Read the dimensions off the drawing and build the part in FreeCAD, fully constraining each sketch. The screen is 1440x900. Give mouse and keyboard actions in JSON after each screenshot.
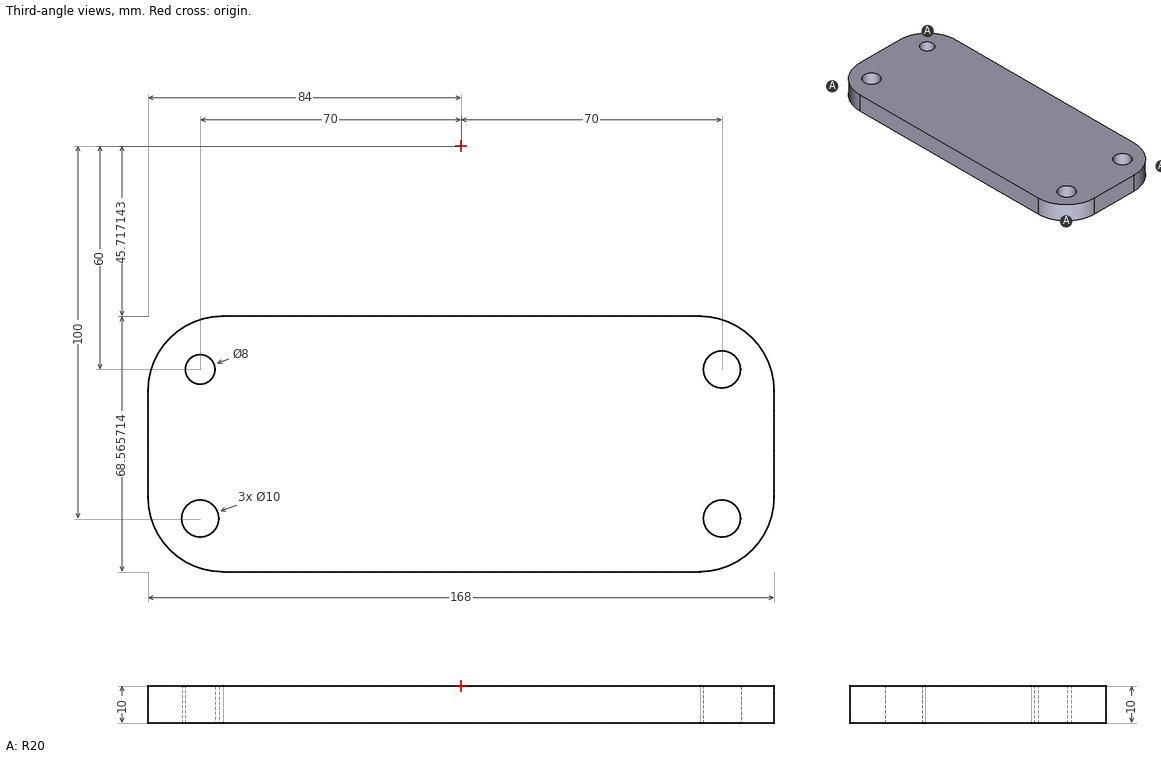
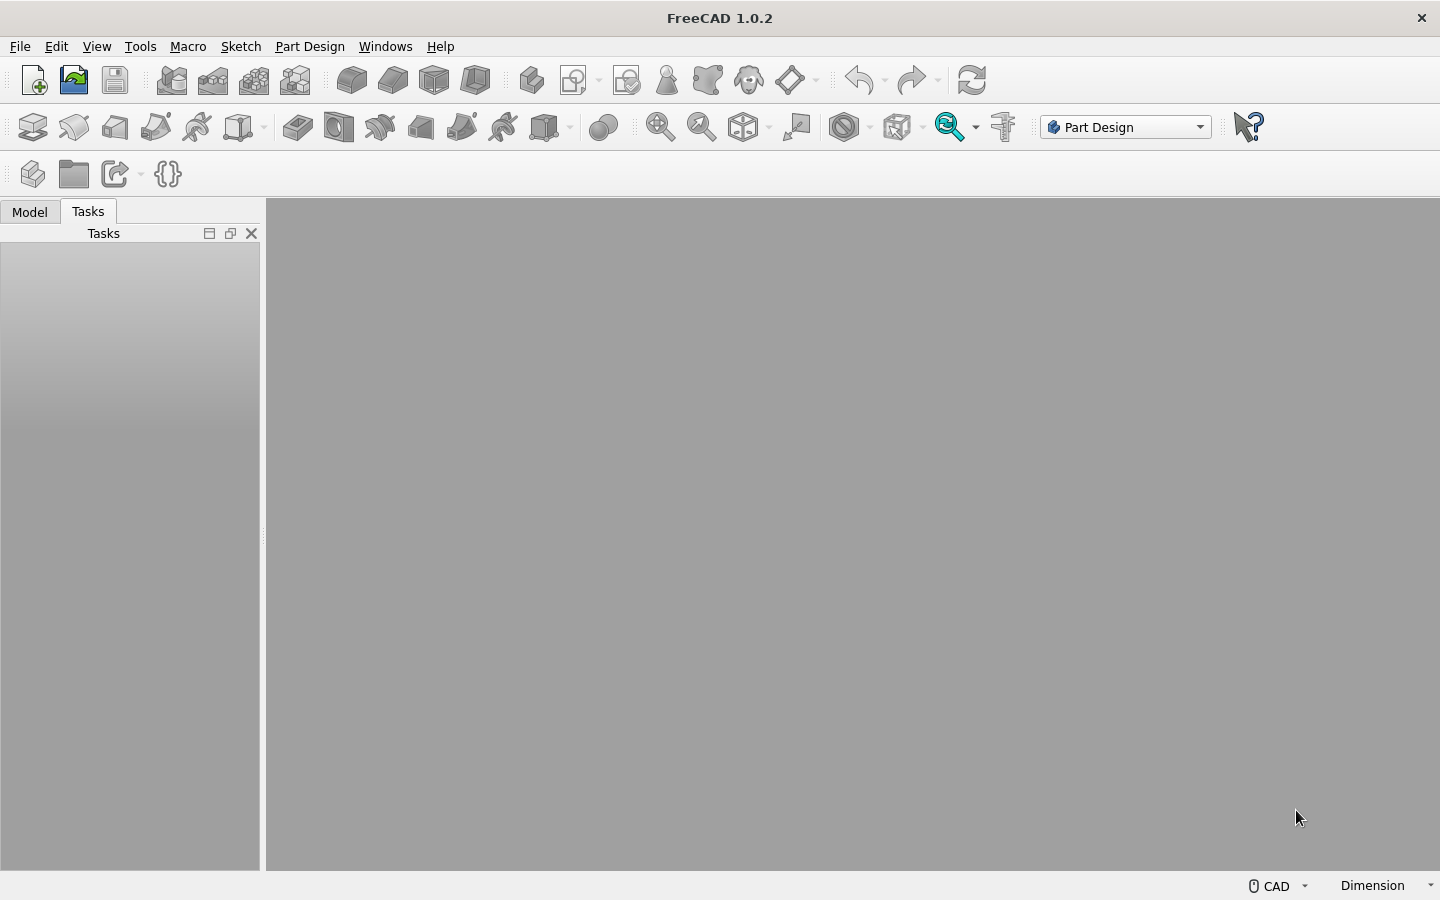
{"action": "left_click", "coordinate": [33, 80]}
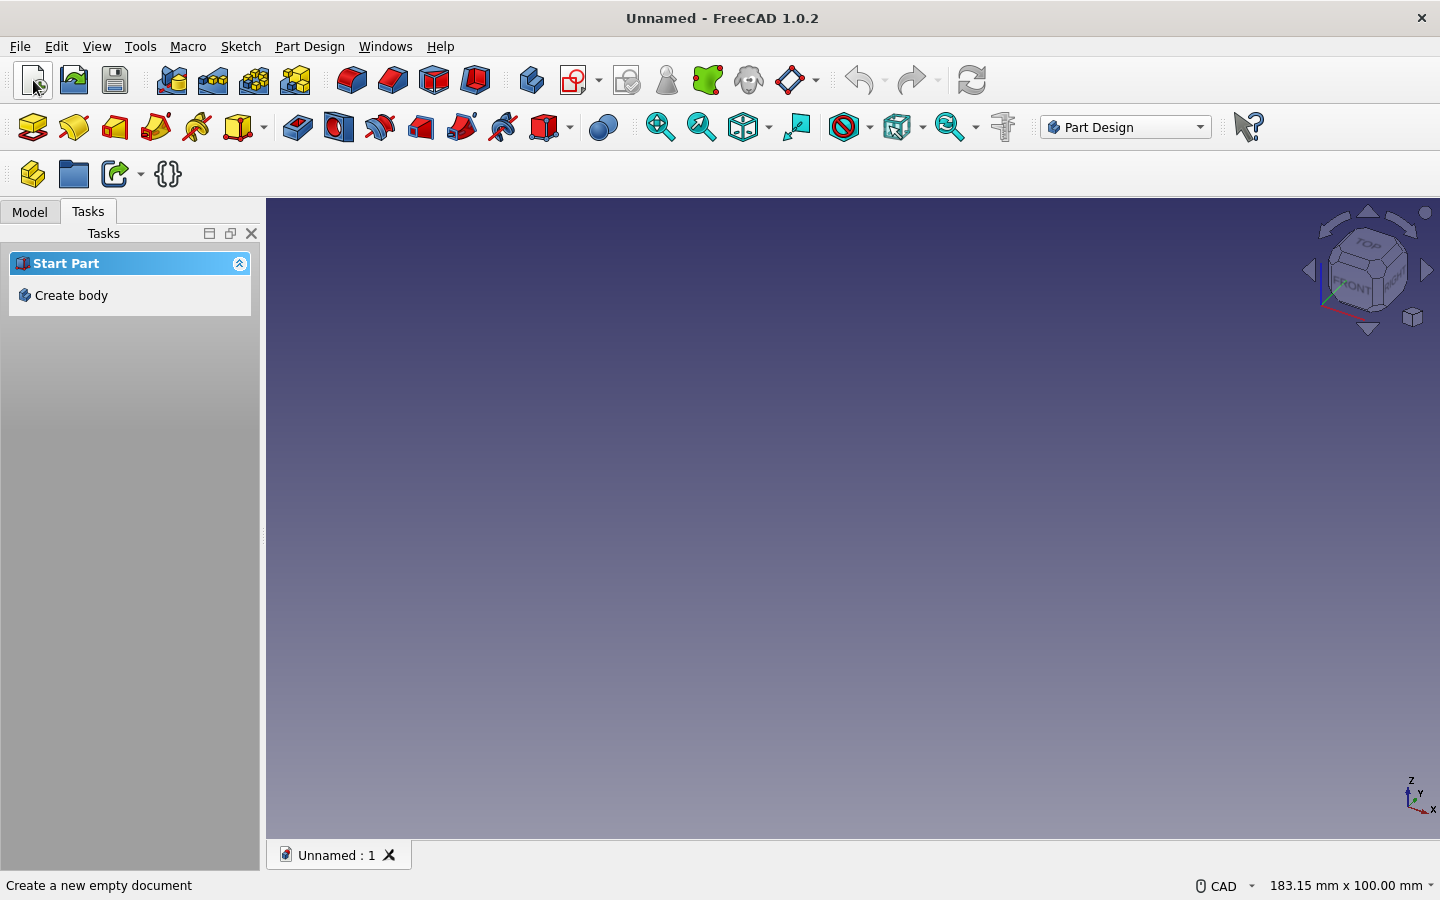
{"action": "left_click", "coordinate": [572, 80]}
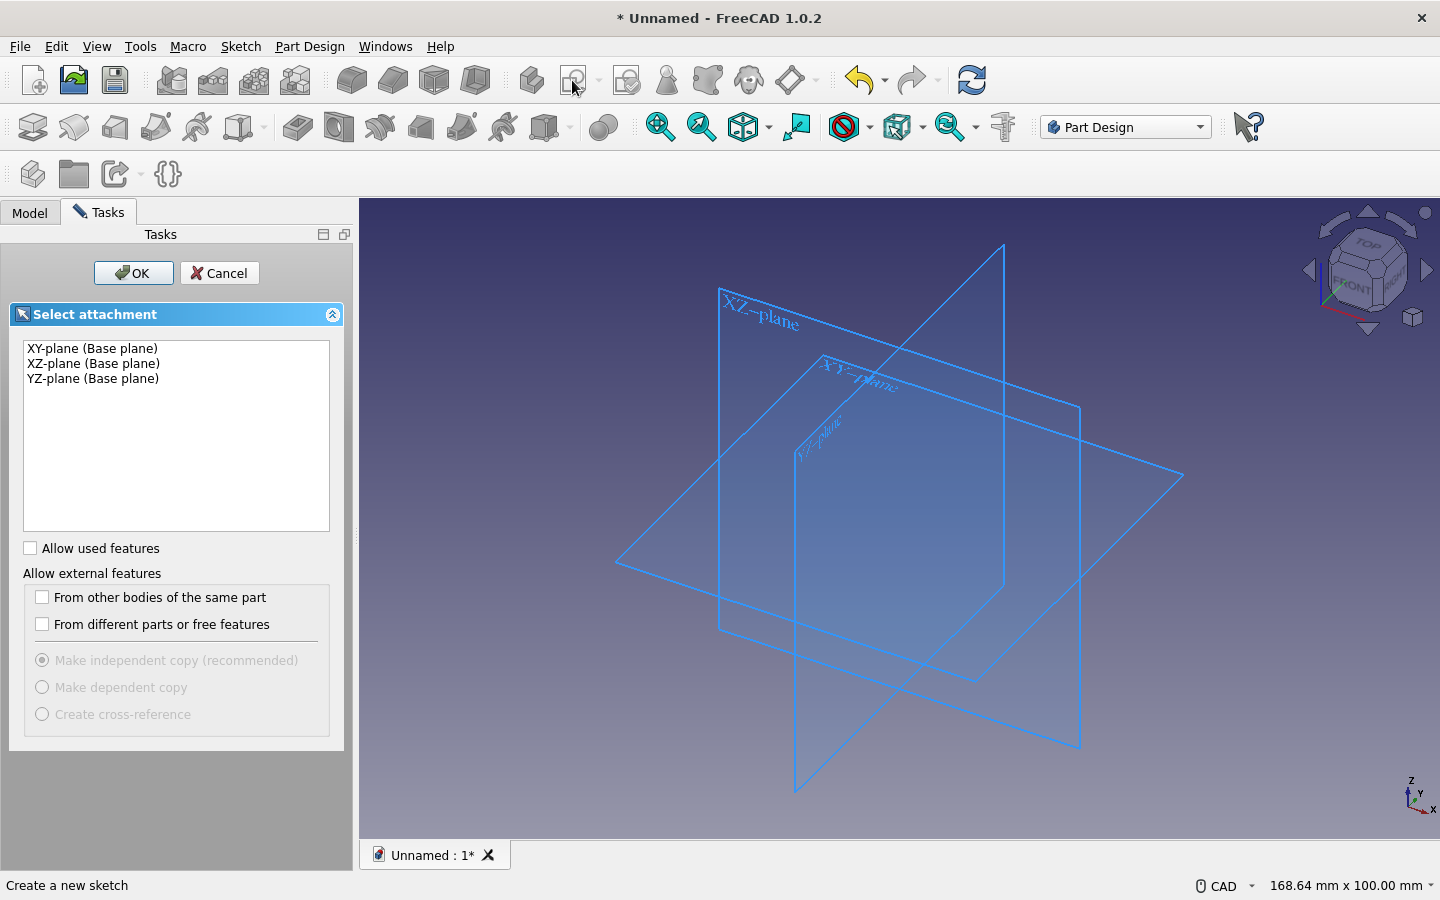
{"action": "left_click", "coordinate": [84, 348]}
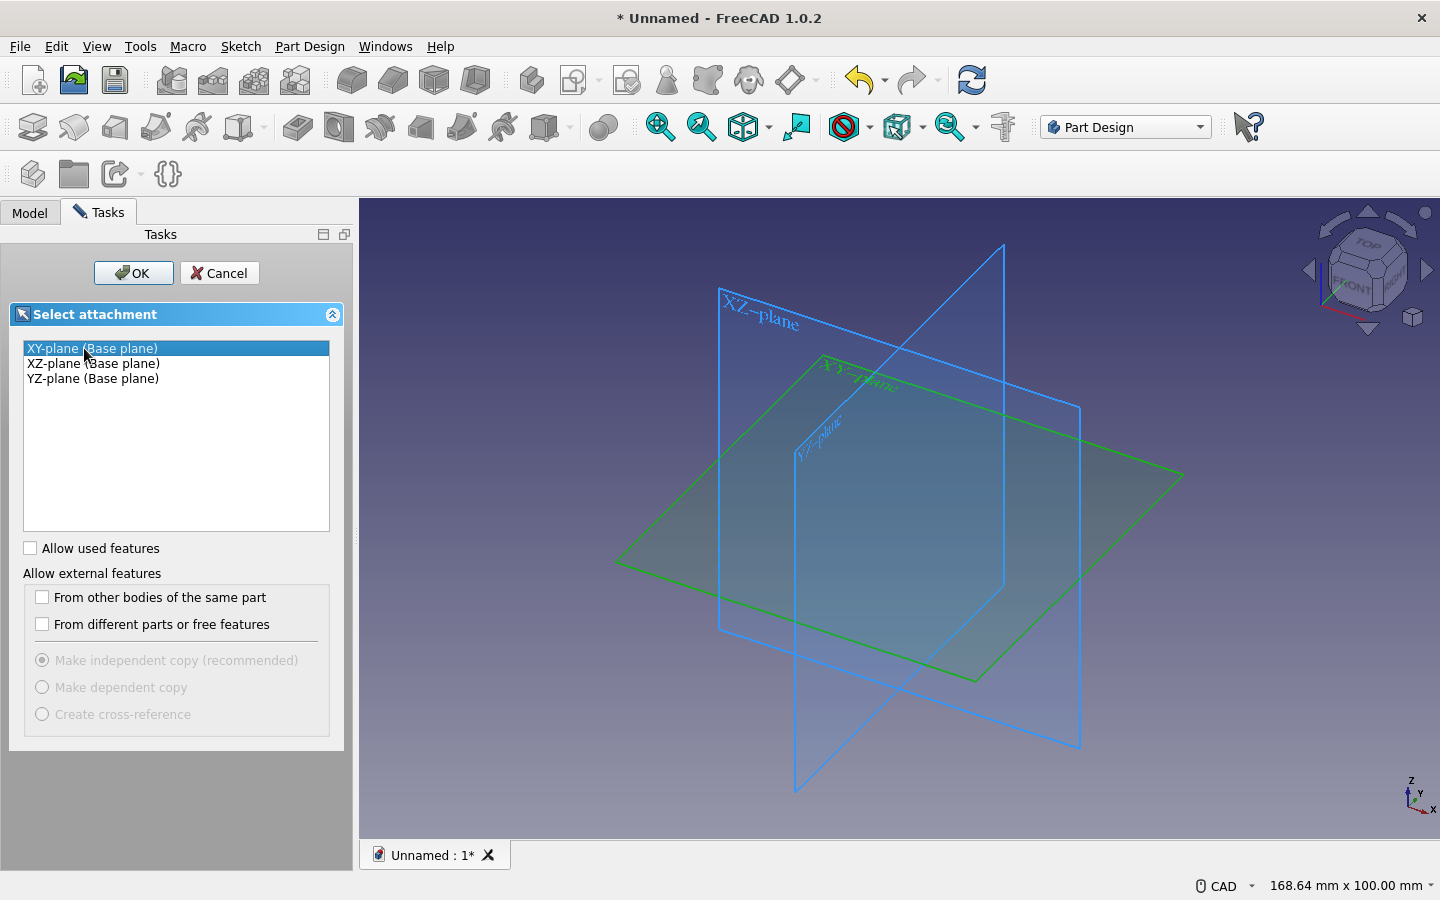
{"action": "left_click", "coordinate": [134, 273]}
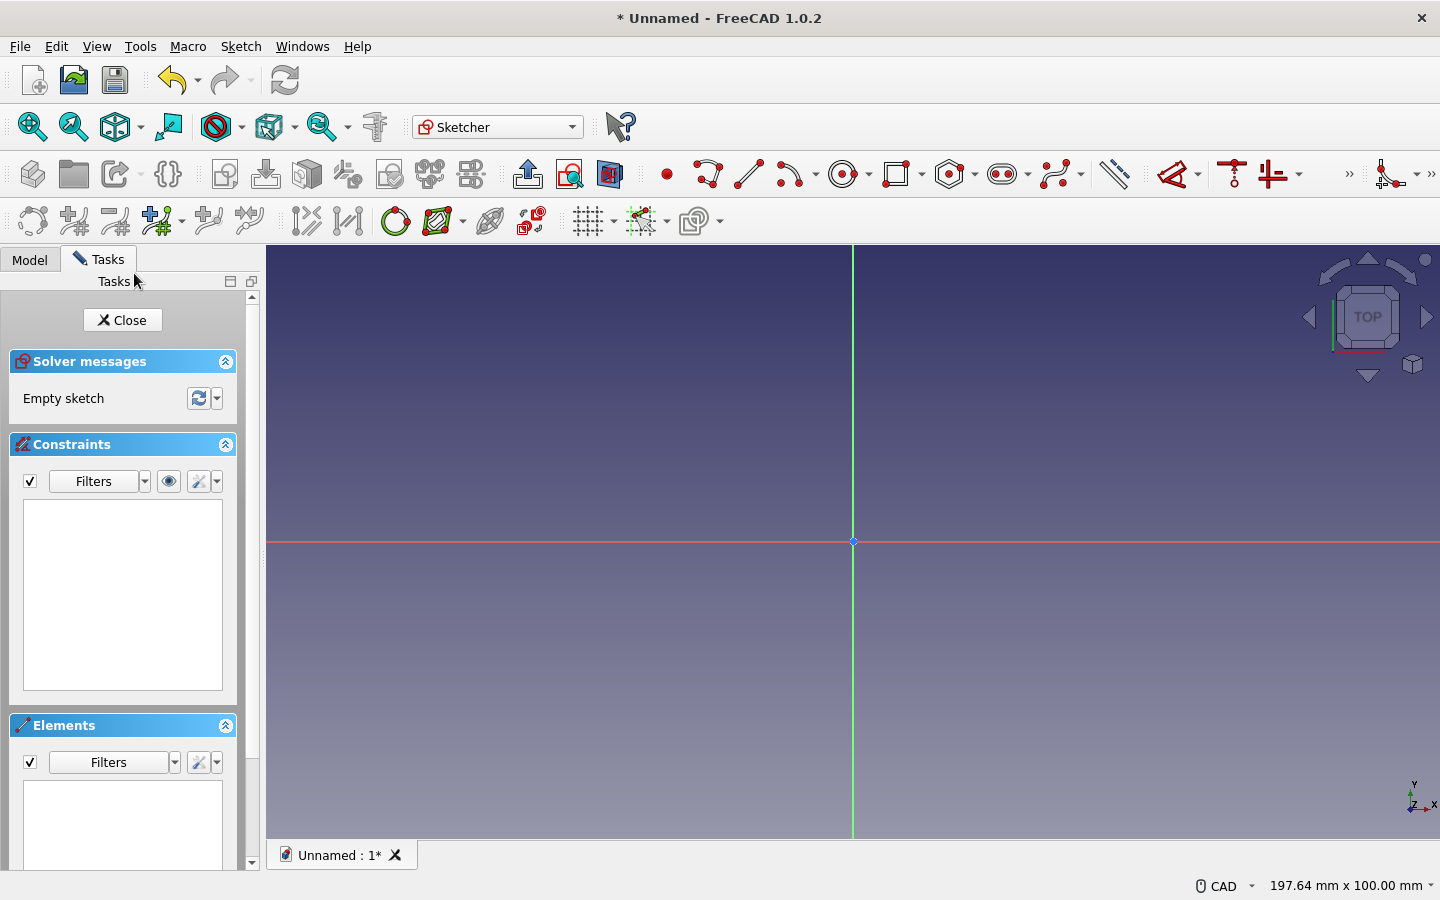
{"action": "scroll", "coordinate": [729, 273], "scroll_direction": "down", "scroll_amount": 4}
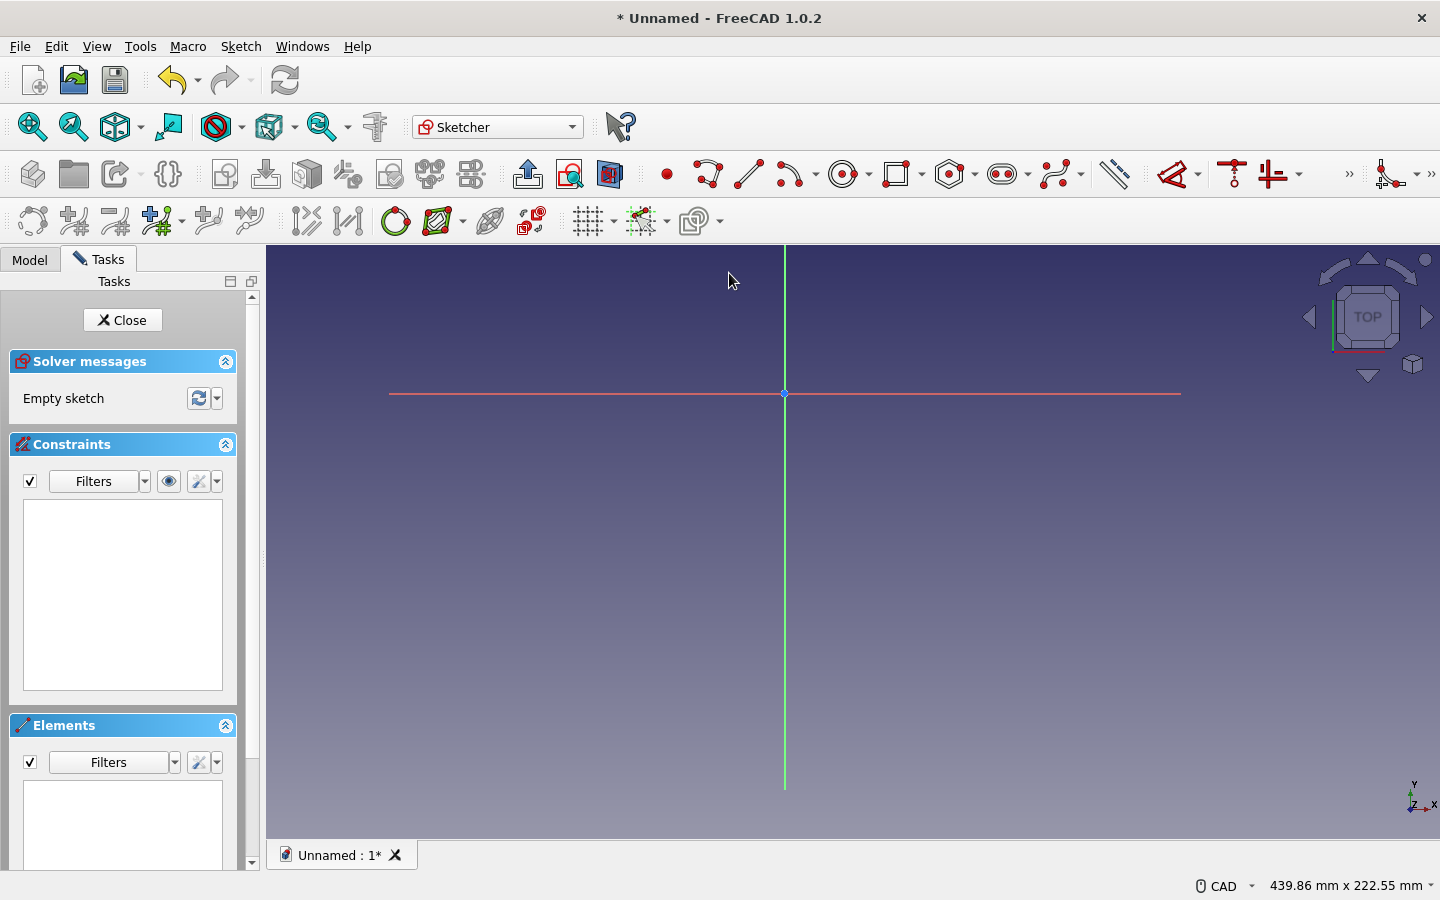
{"action": "left_click", "coordinate": [896, 174]}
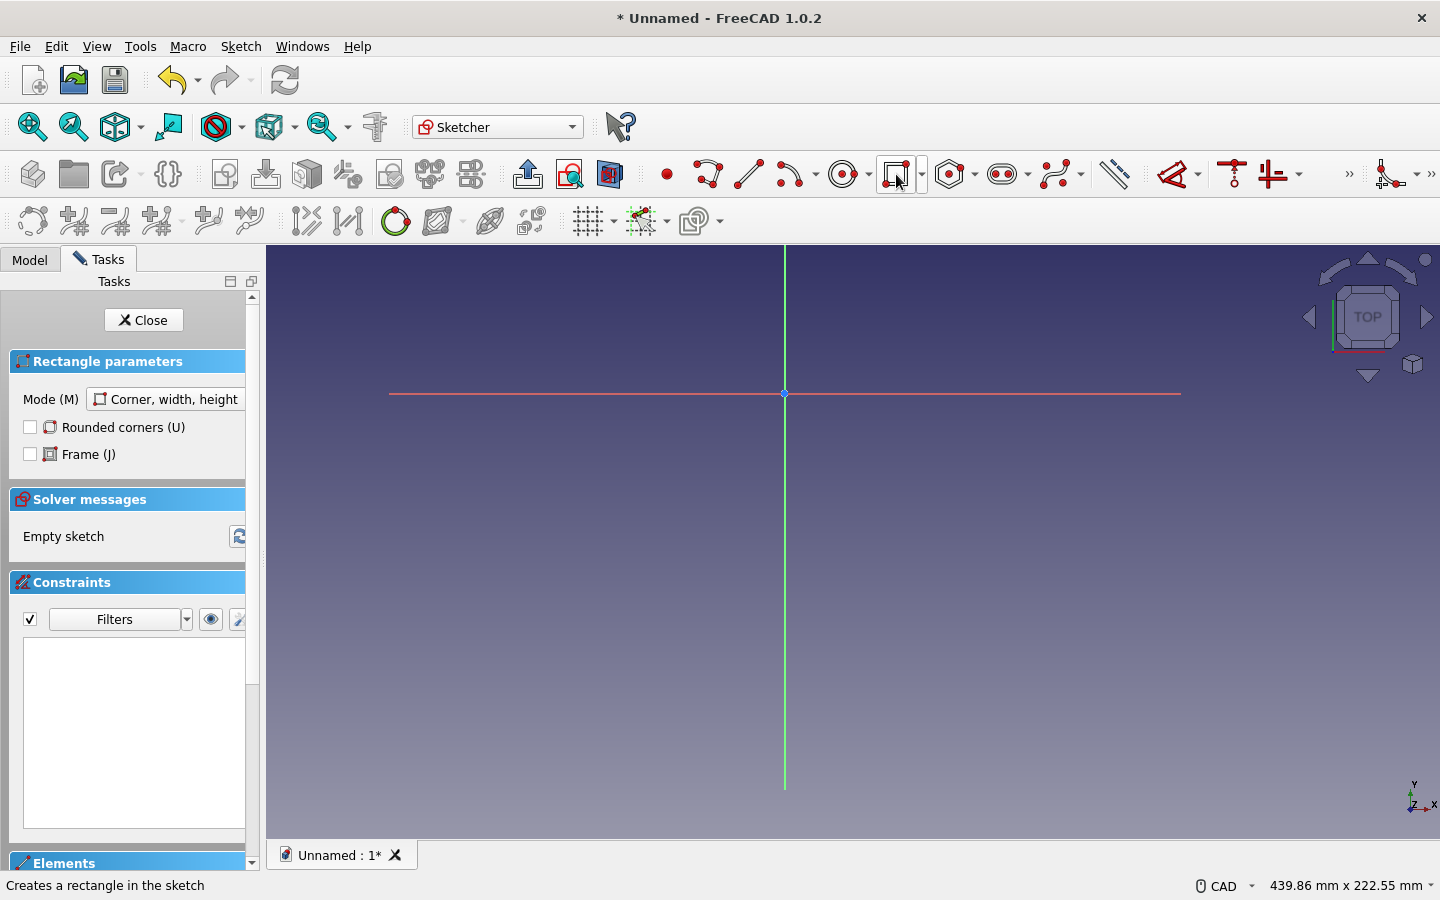
{"action": "left_click", "coordinate": [561, 516]}
{"action": "left_click", "coordinate": [1009, 699]}
{"action": "key", "text": "Escape"}